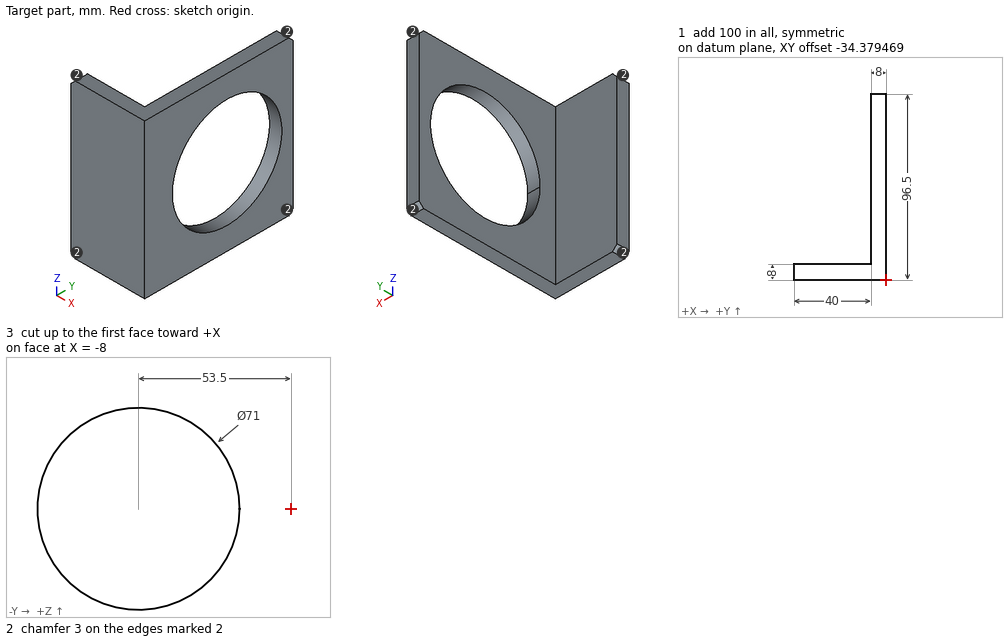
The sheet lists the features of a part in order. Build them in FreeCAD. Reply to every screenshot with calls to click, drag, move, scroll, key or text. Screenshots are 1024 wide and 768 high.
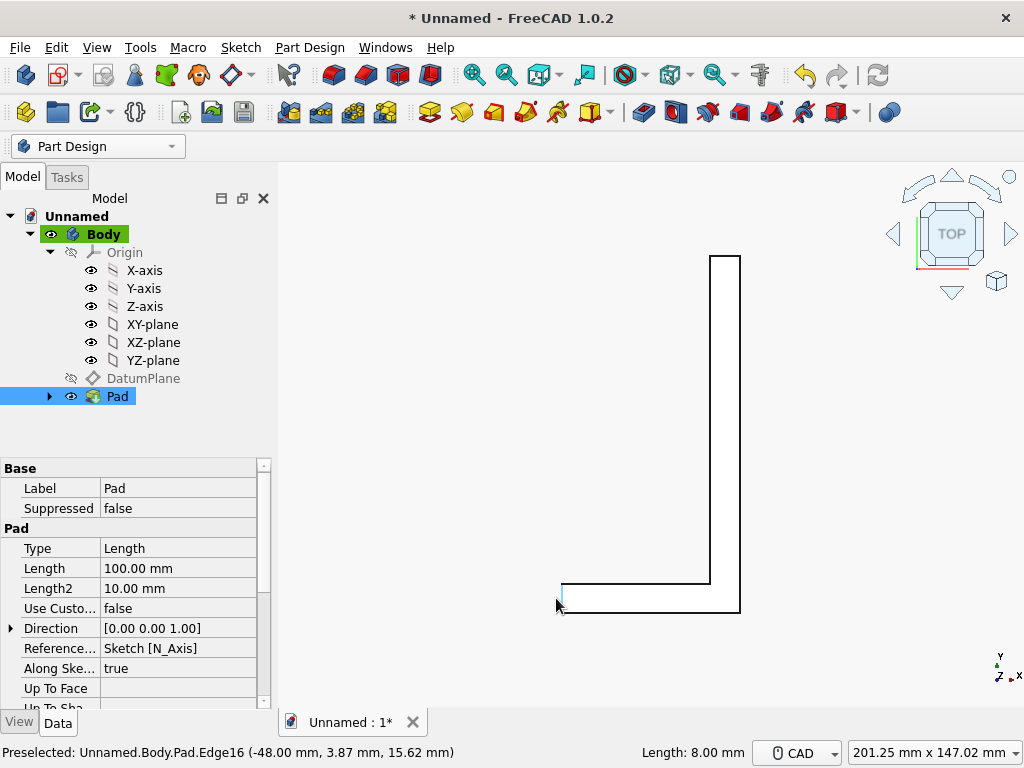
click(725, 255, ctrl)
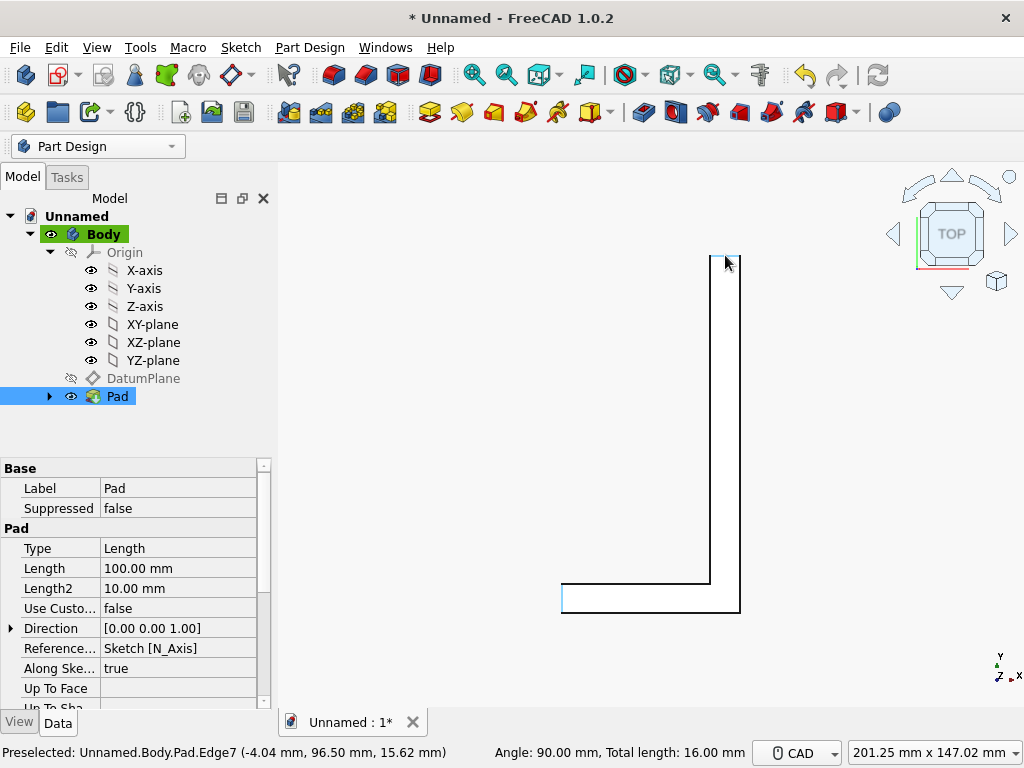
key(1)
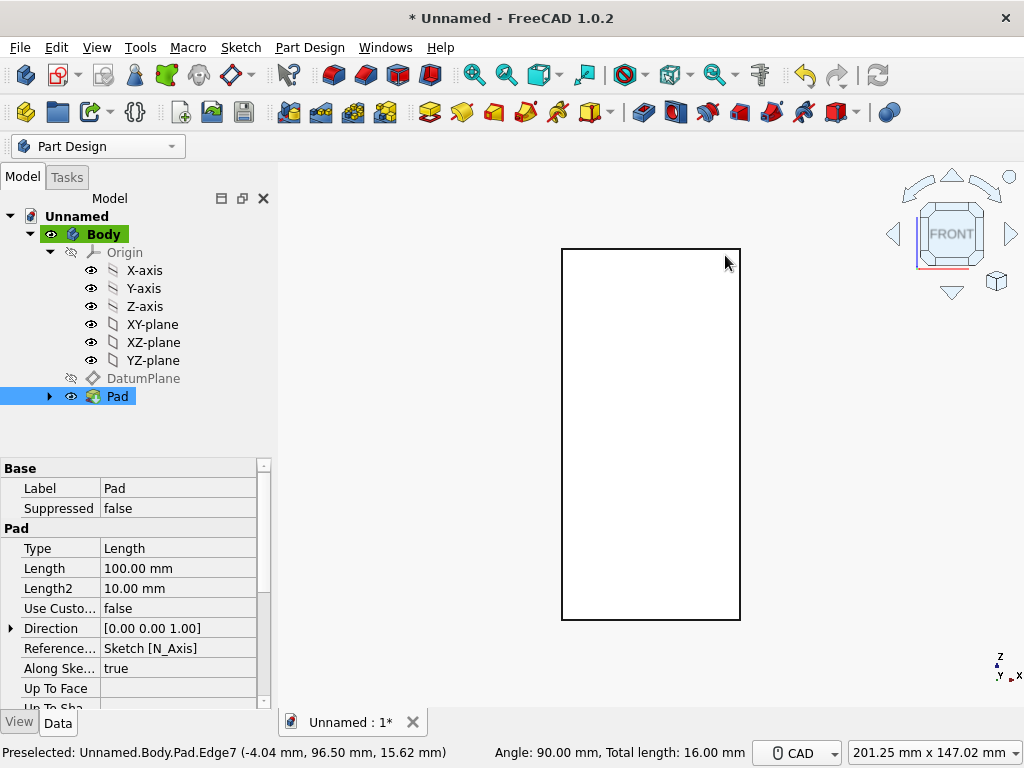
key(3)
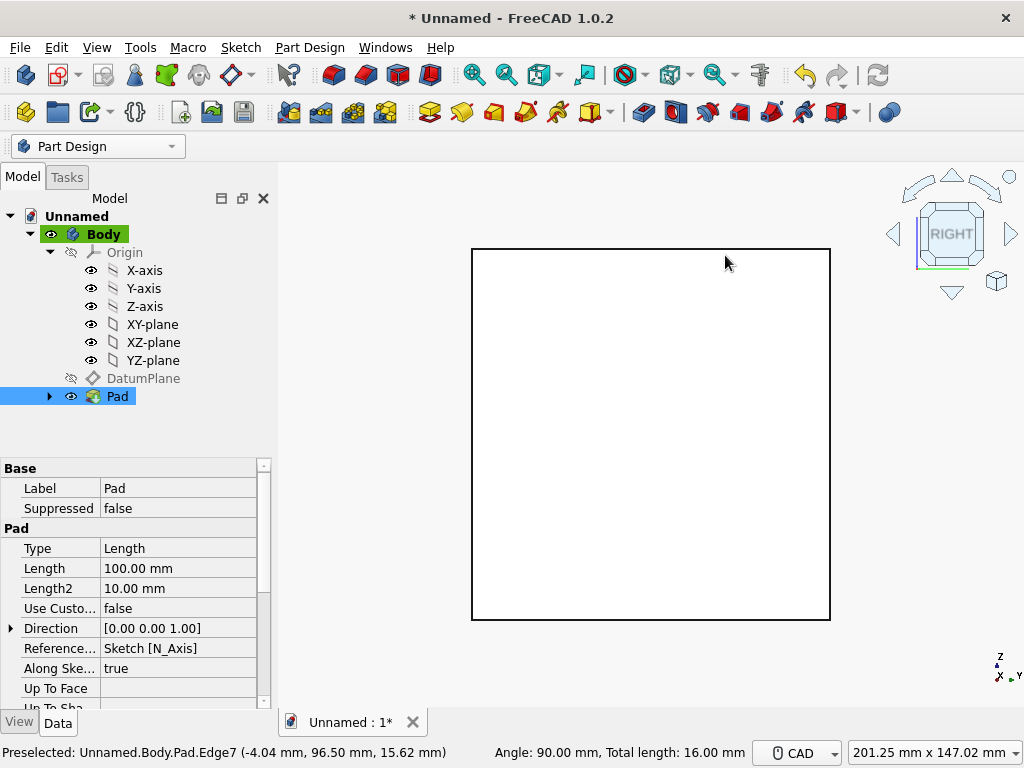
key(5)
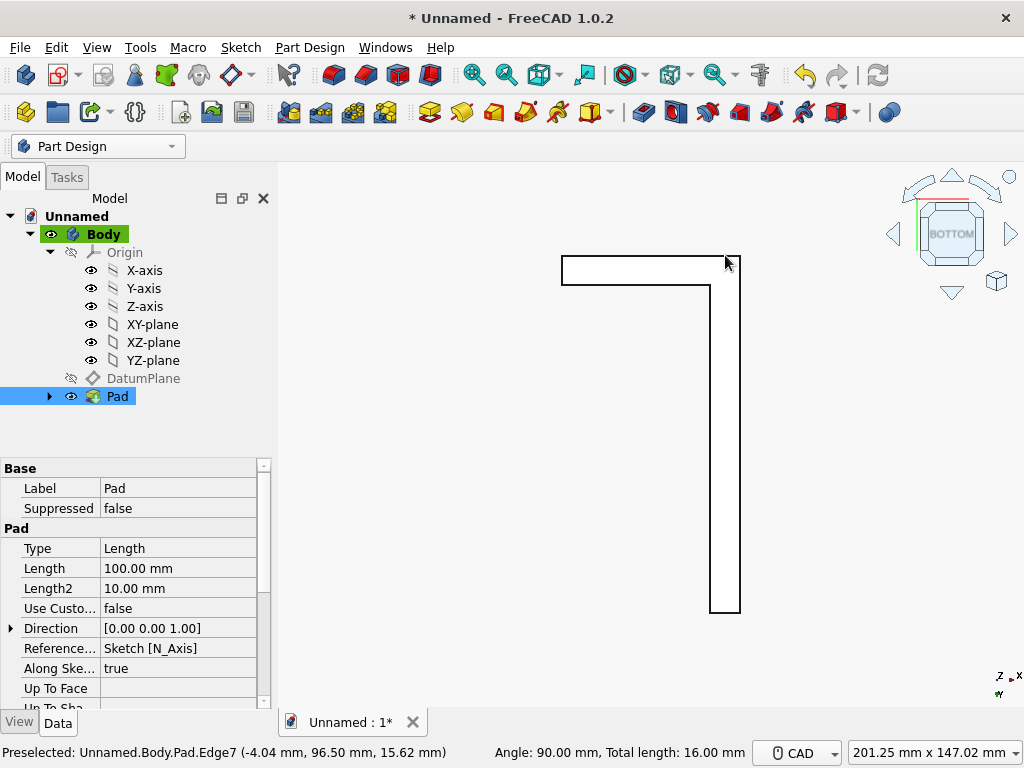
click(562, 269, ctrl)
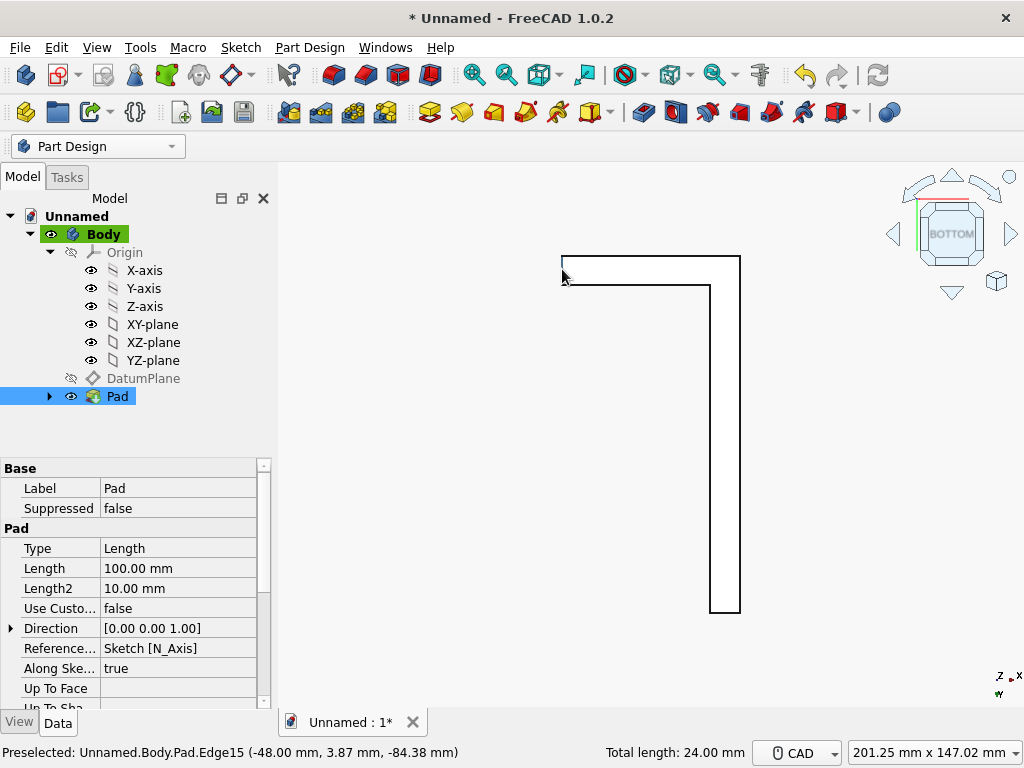
click(725, 612, ctrl)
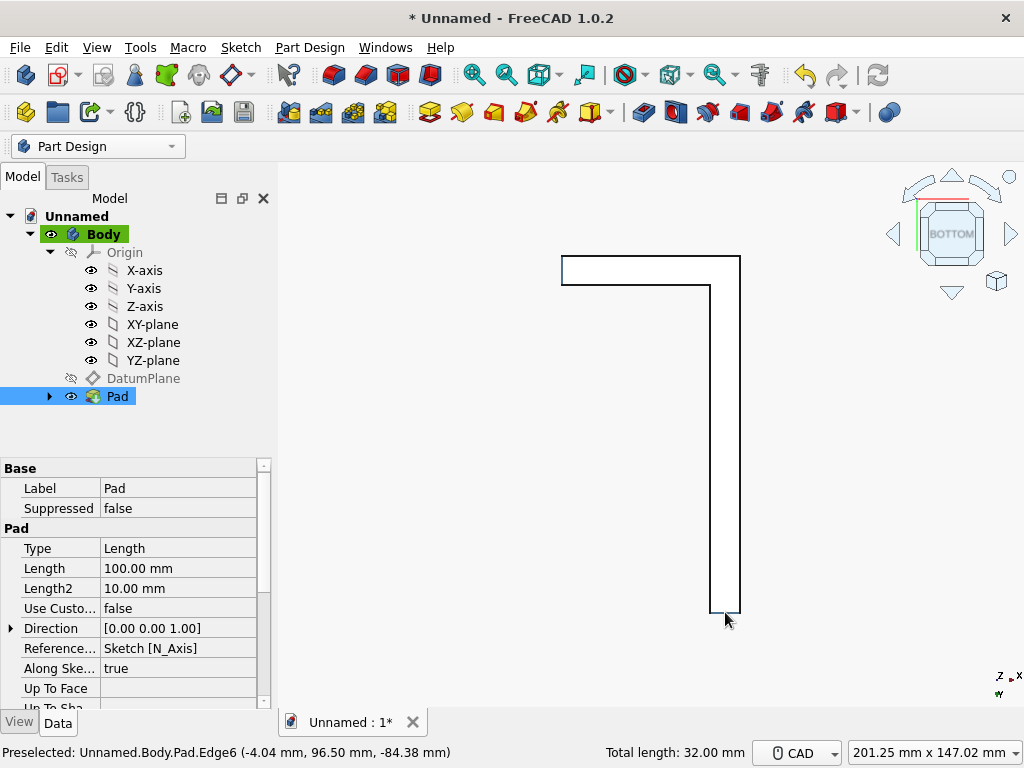
click(366, 76)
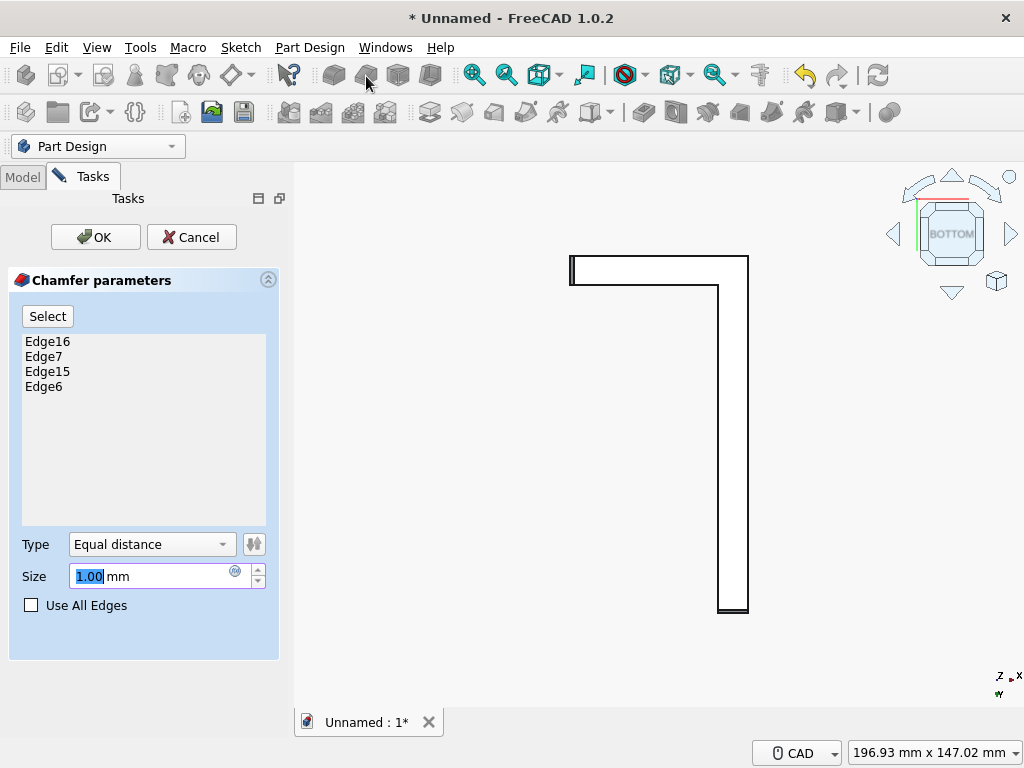
text(3)
key(Tab)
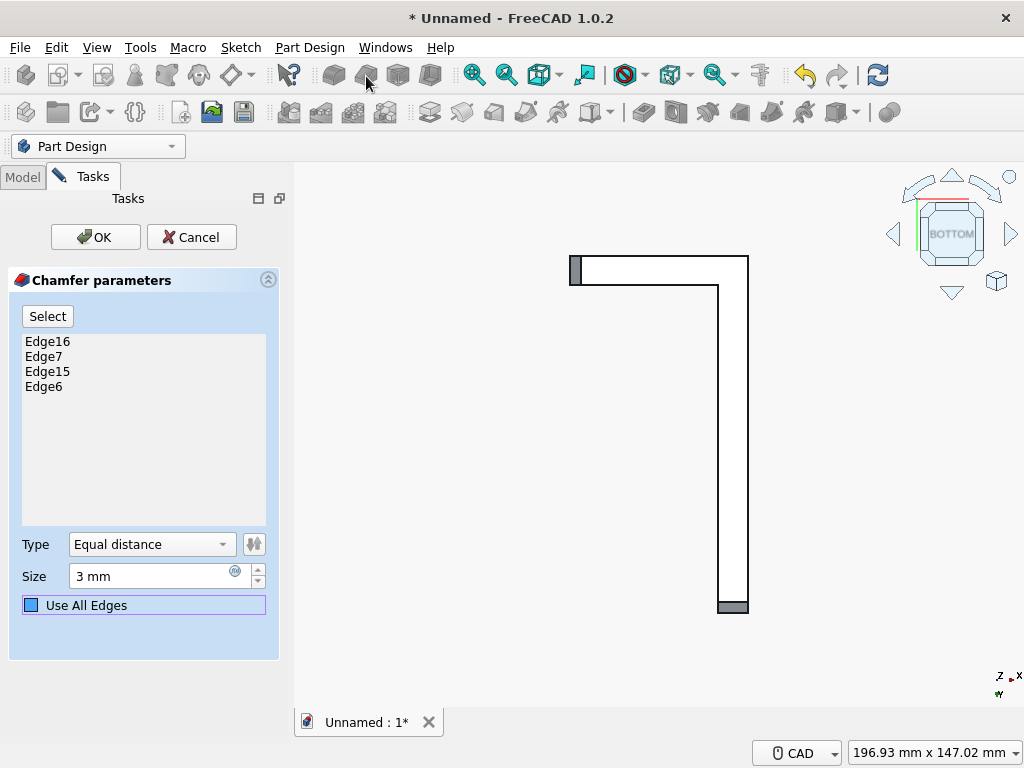
click(96, 237)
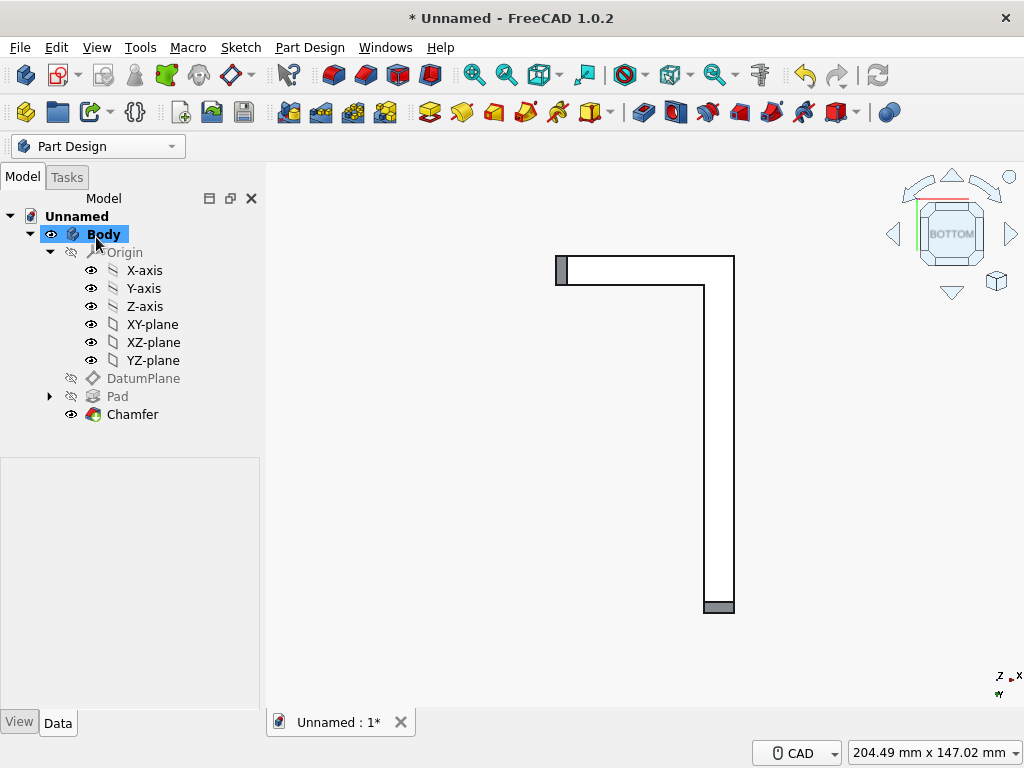
key(6)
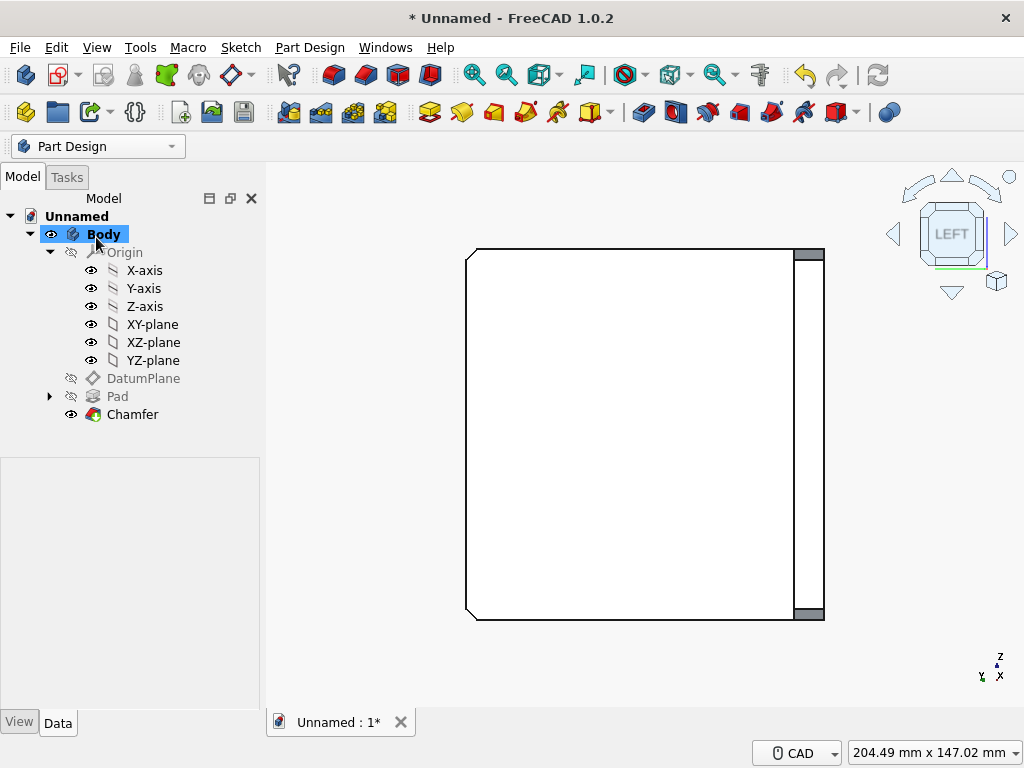
click(630, 433)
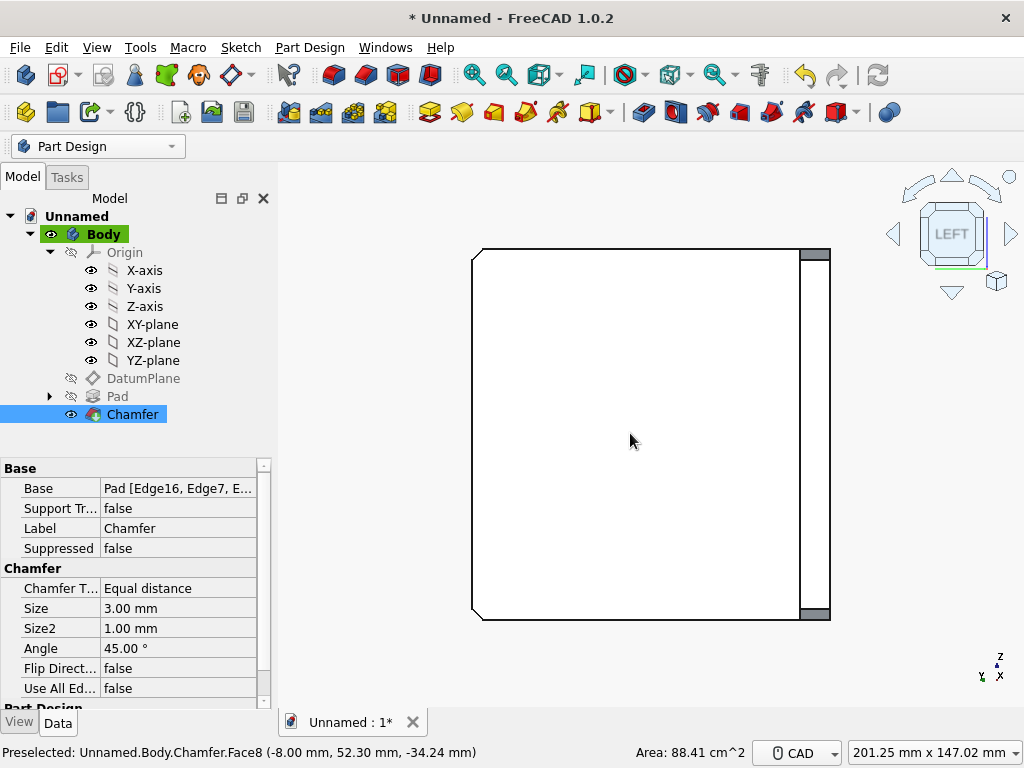
click(58, 76)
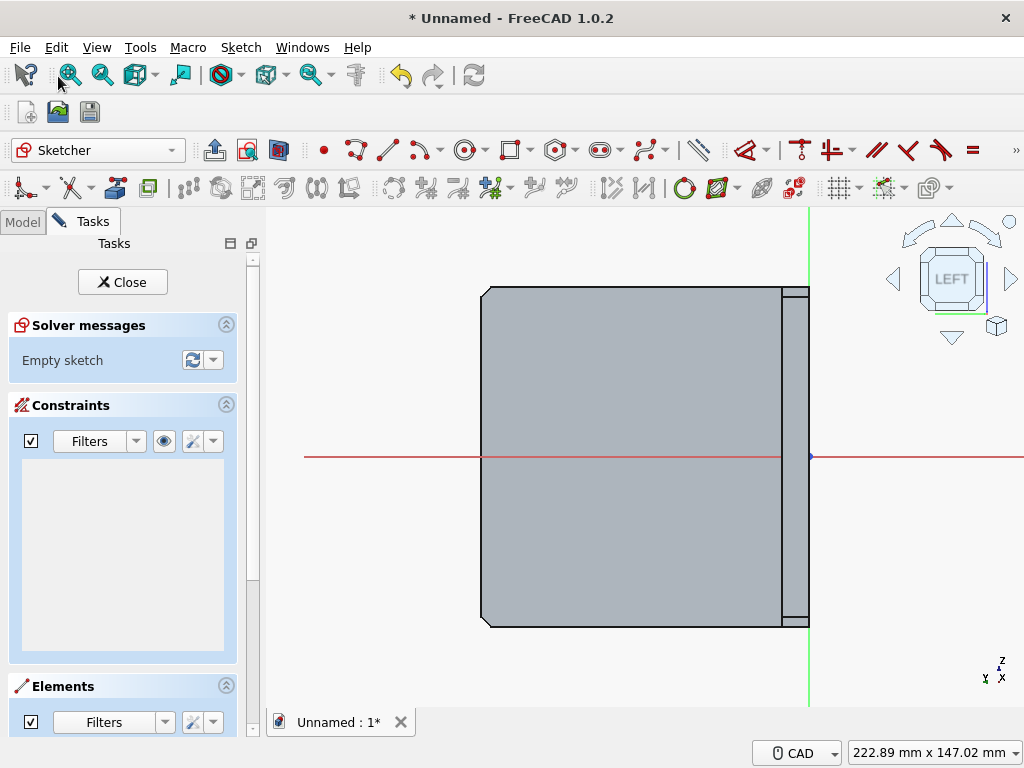
key(g)
key(c)